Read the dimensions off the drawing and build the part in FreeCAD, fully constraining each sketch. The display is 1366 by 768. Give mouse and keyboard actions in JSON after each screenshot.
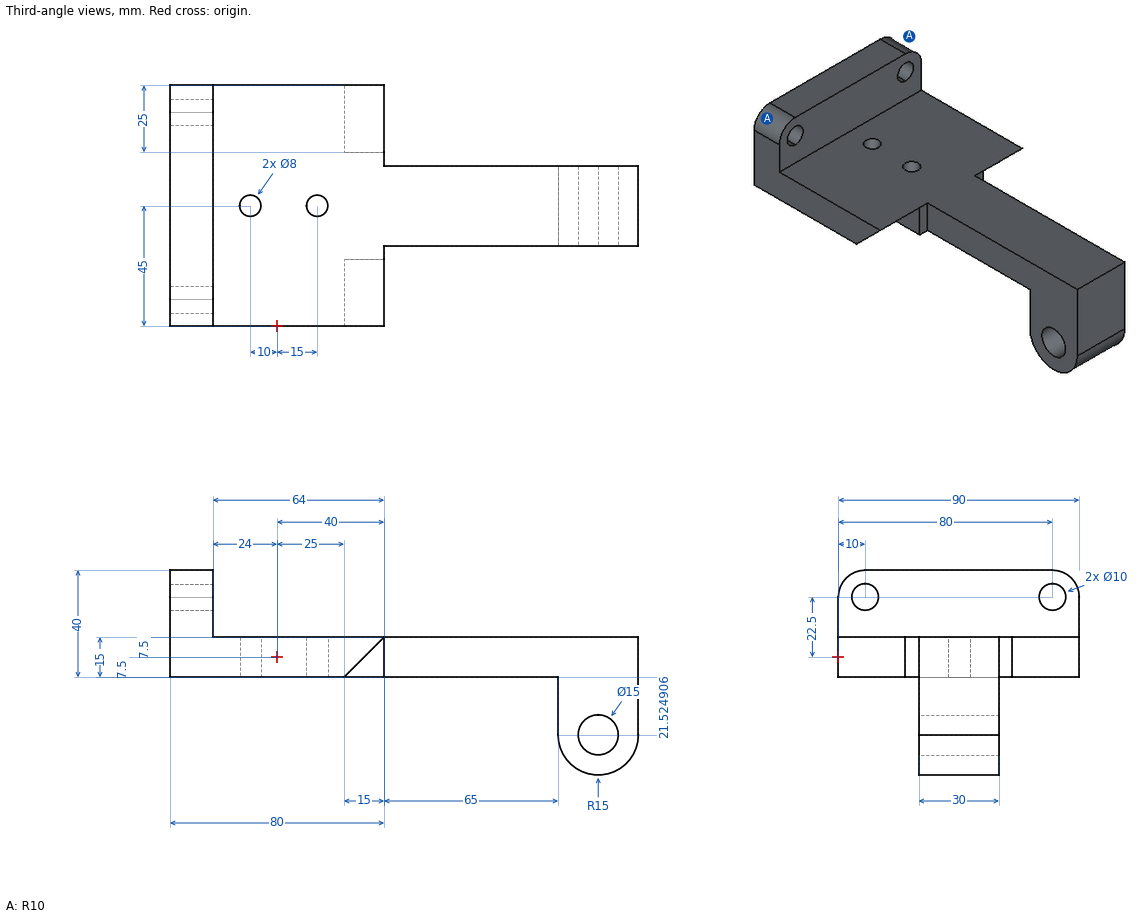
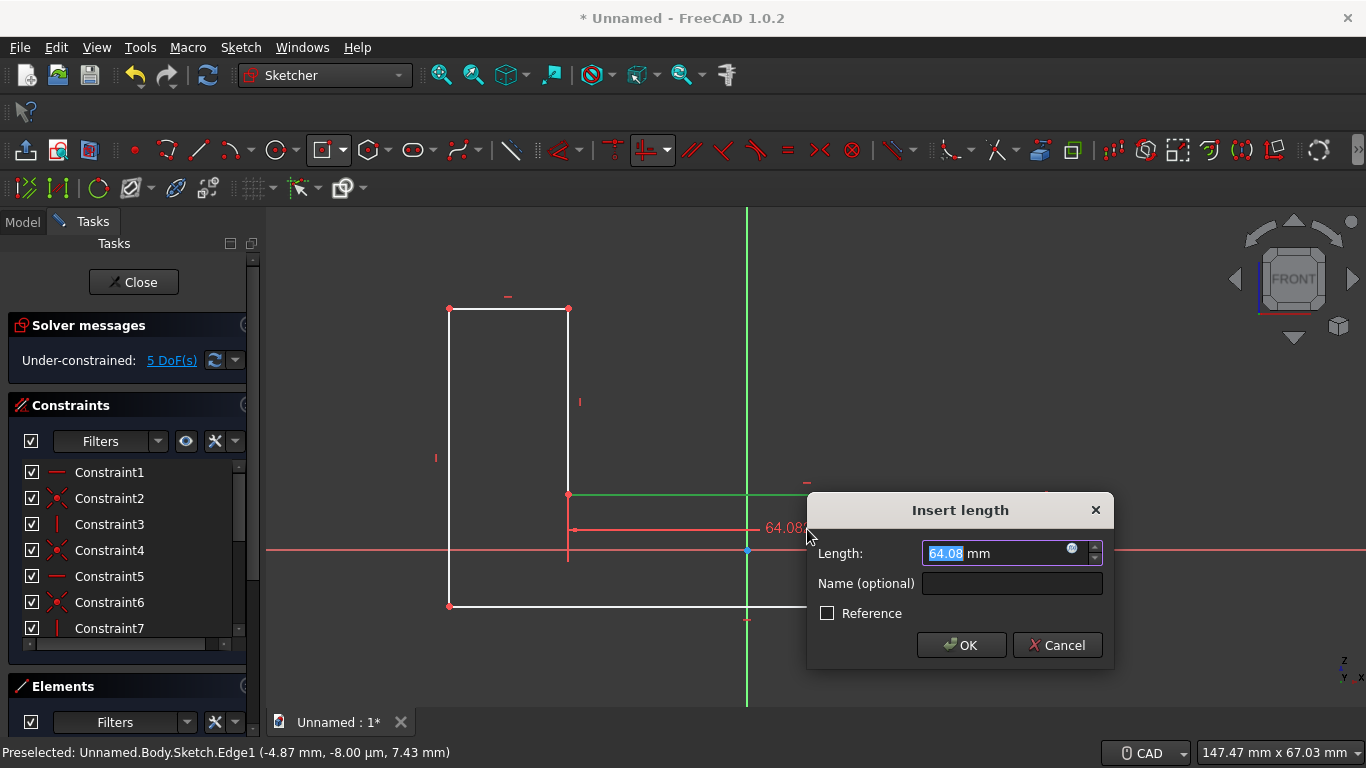
{"action": "type", "text": "64"}
{"action": "key", "text": "Return"}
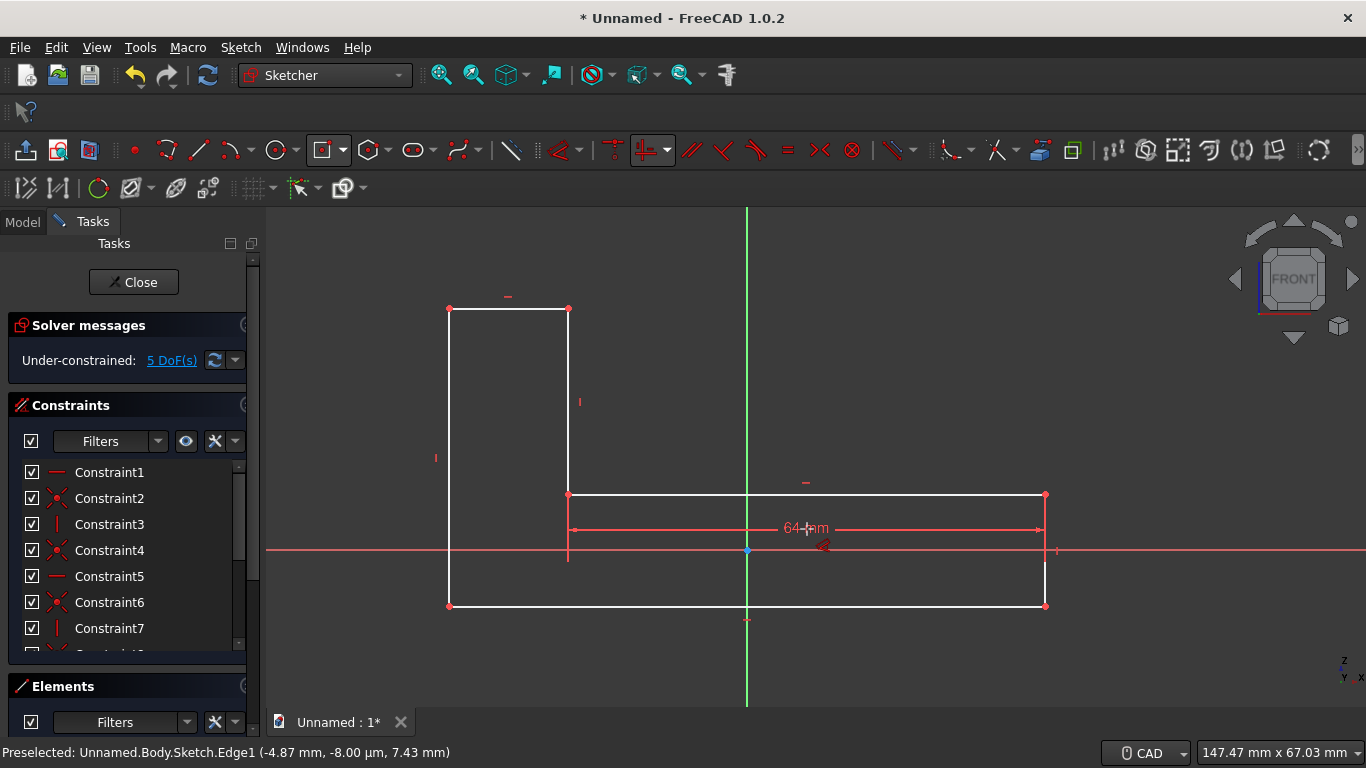
{"action": "left_click", "coordinate": [1045, 529]}
{"action": "left_click", "coordinate": [1079, 525]}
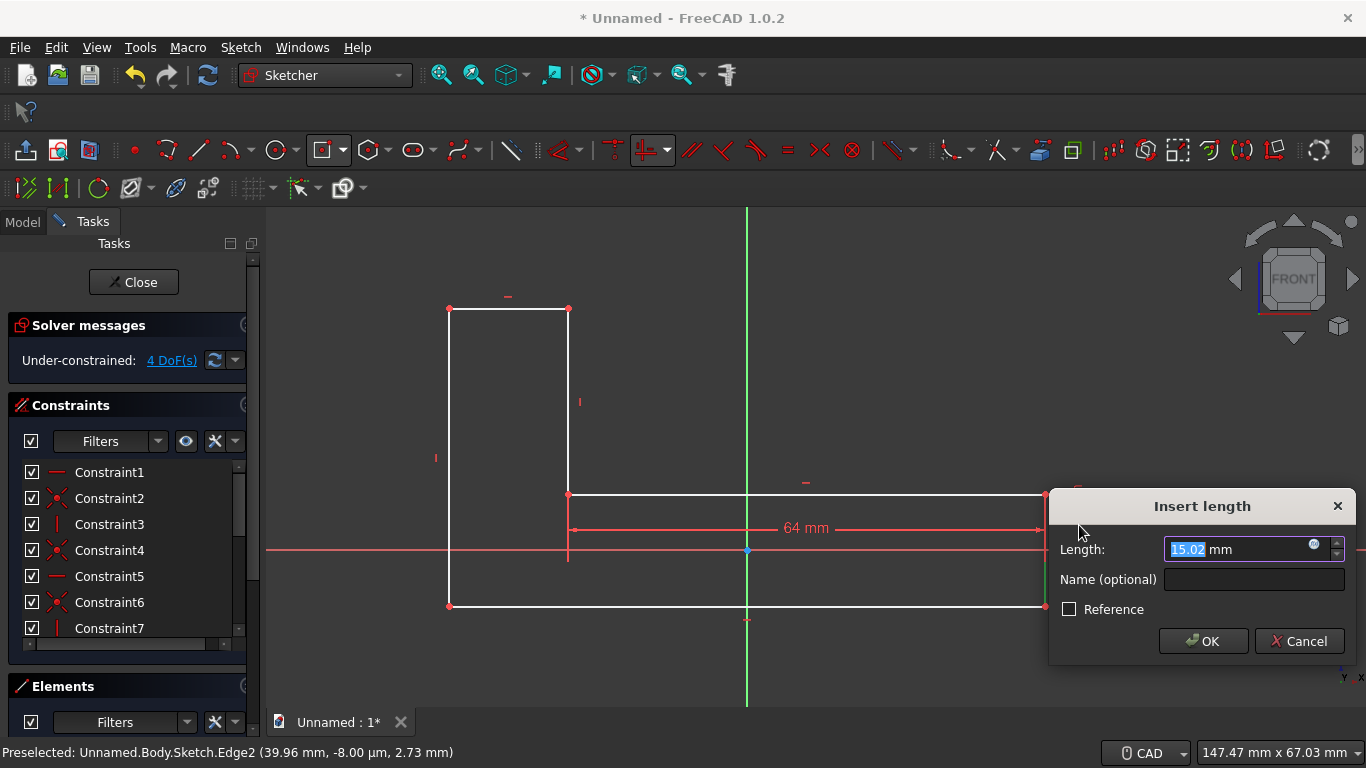
{"action": "type", "text": "15"}
{"action": "key", "text": "Return"}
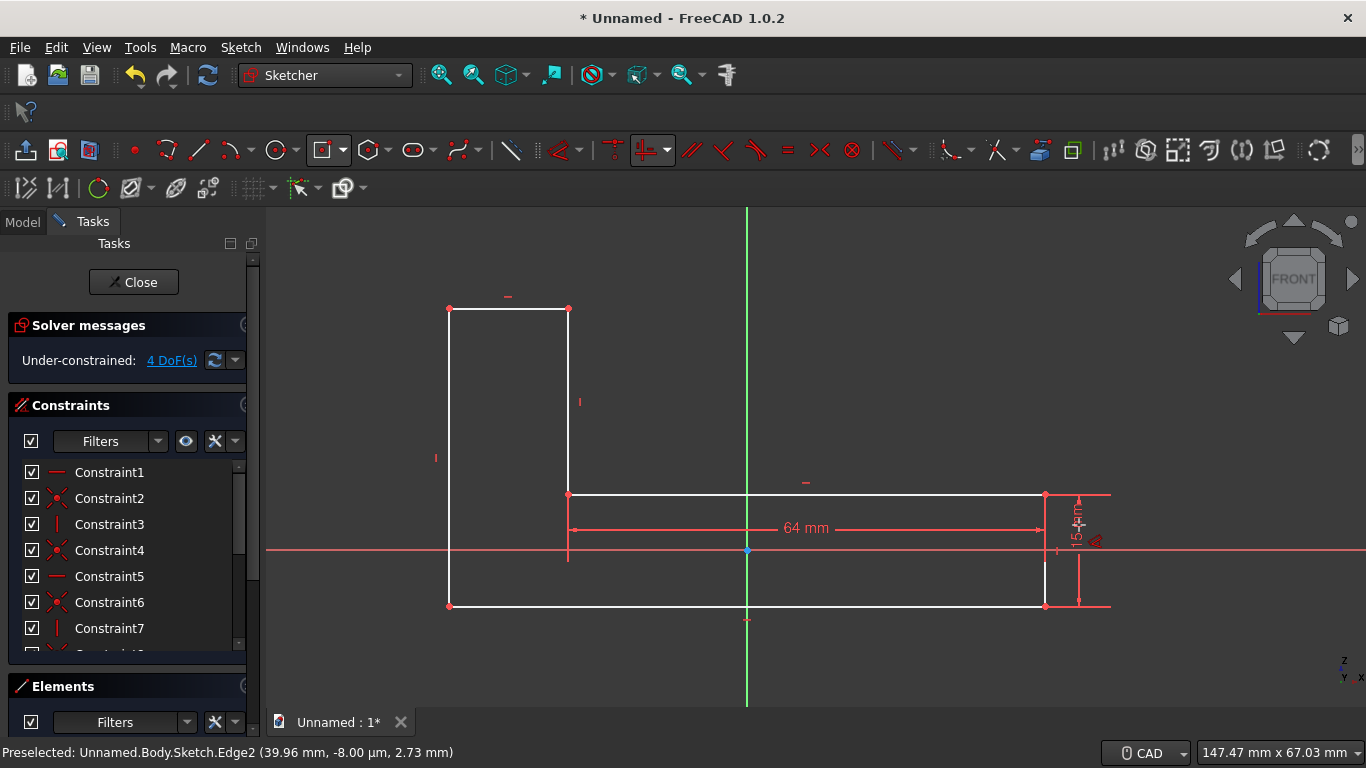
{"action": "left_click", "coordinate": [866, 607]}
{"action": "left_click", "coordinate": [610, 641]}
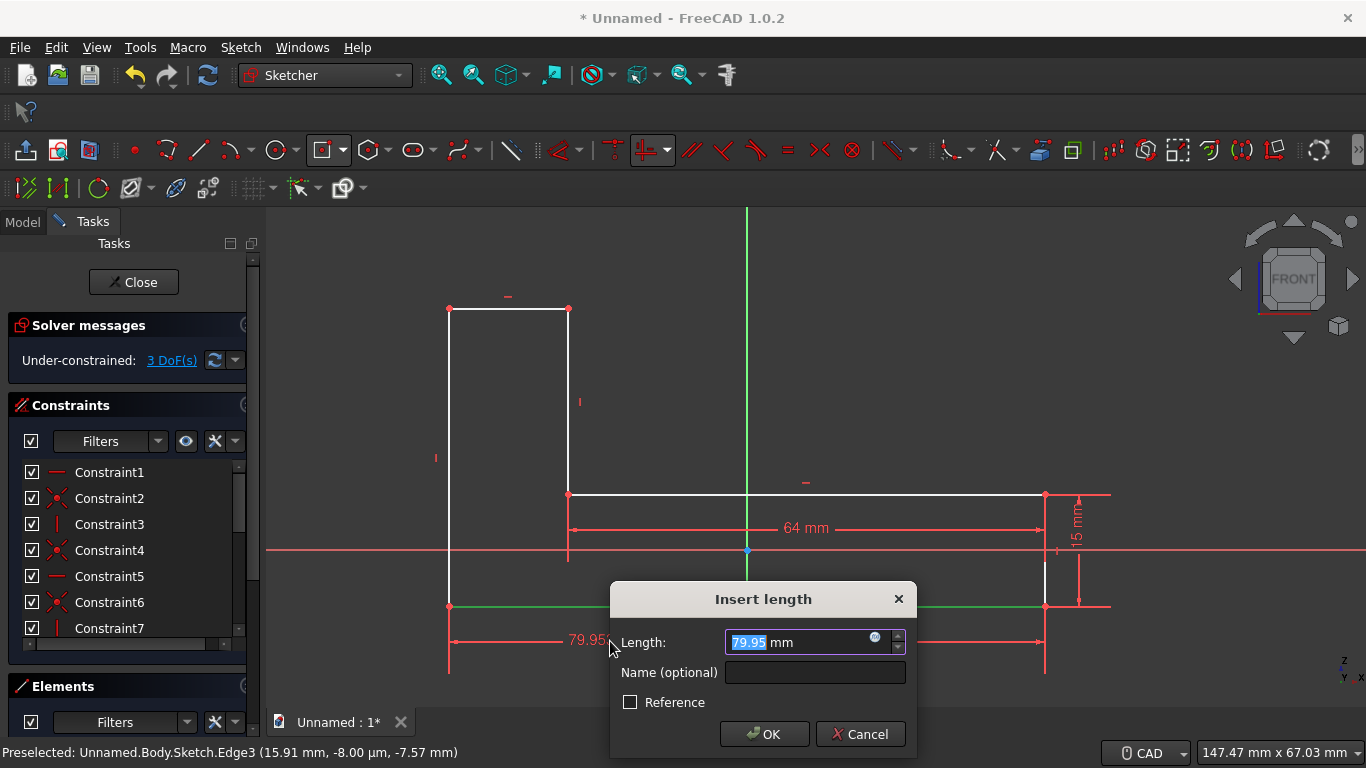
{"action": "type", "text": "80"}
{"action": "key", "text": "Return"}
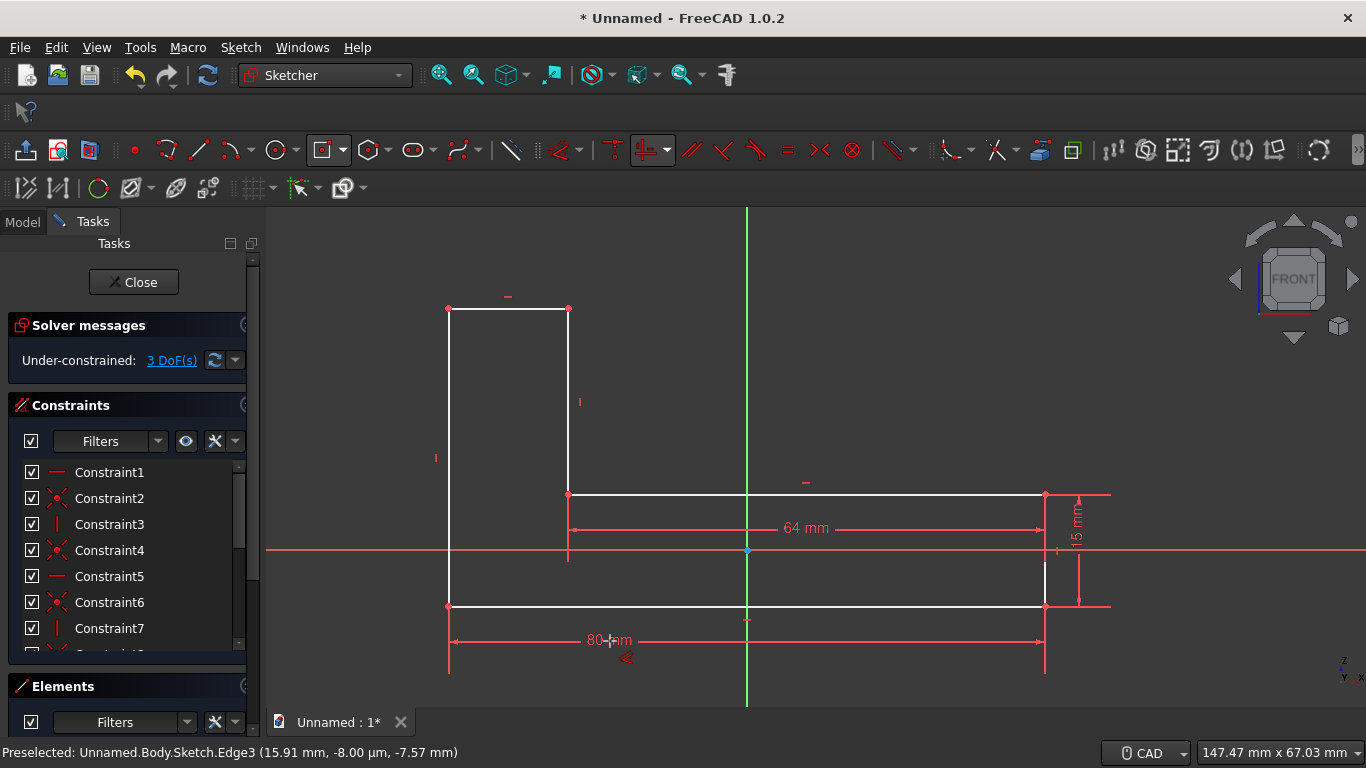
{"action": "left_click", "coordinate": [449, 518]}
{"action": "left_click", "coordinate": [415, 458]}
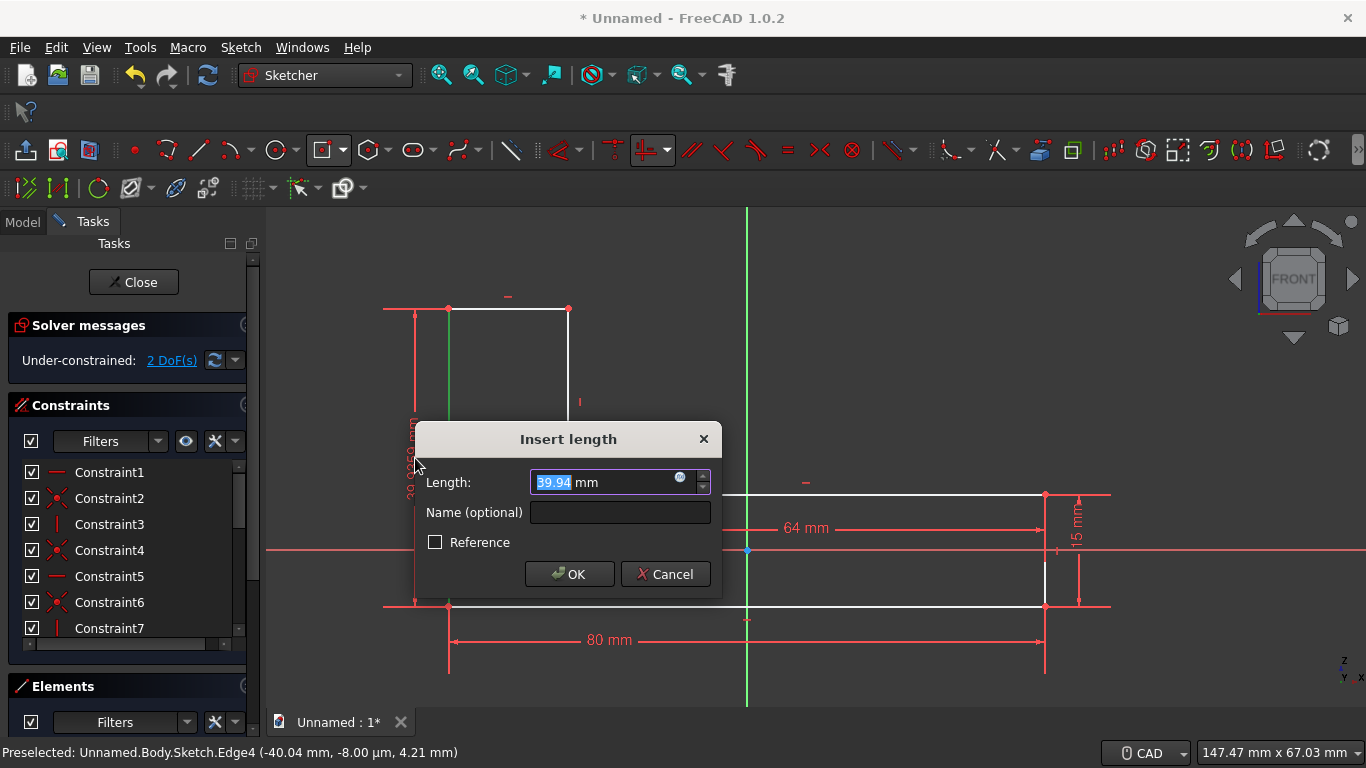
{"action": "type", "text": "40"}
{"action": "key", "text": "Return"}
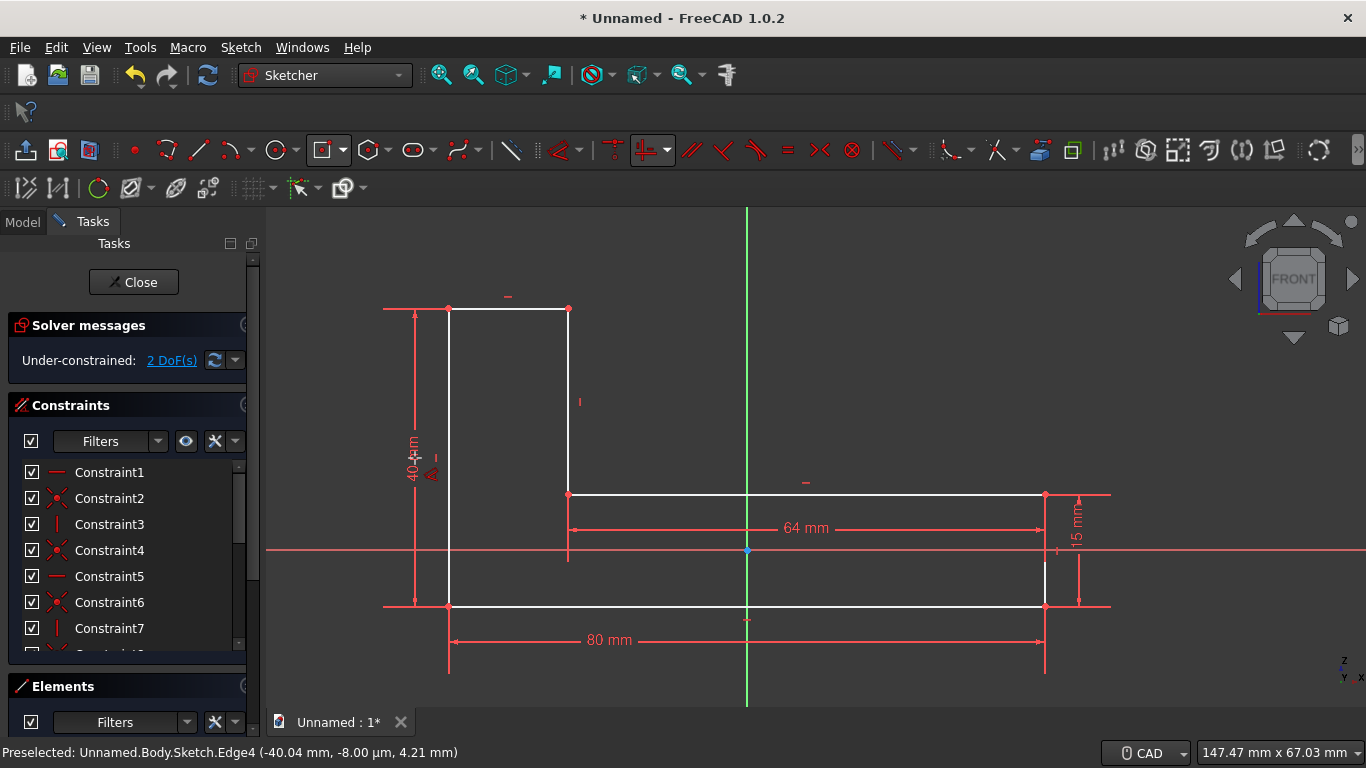
{"action": "left_click", "coordinate": [568, 495]}
{"action": "left_click", "coordinate": [658, 584]}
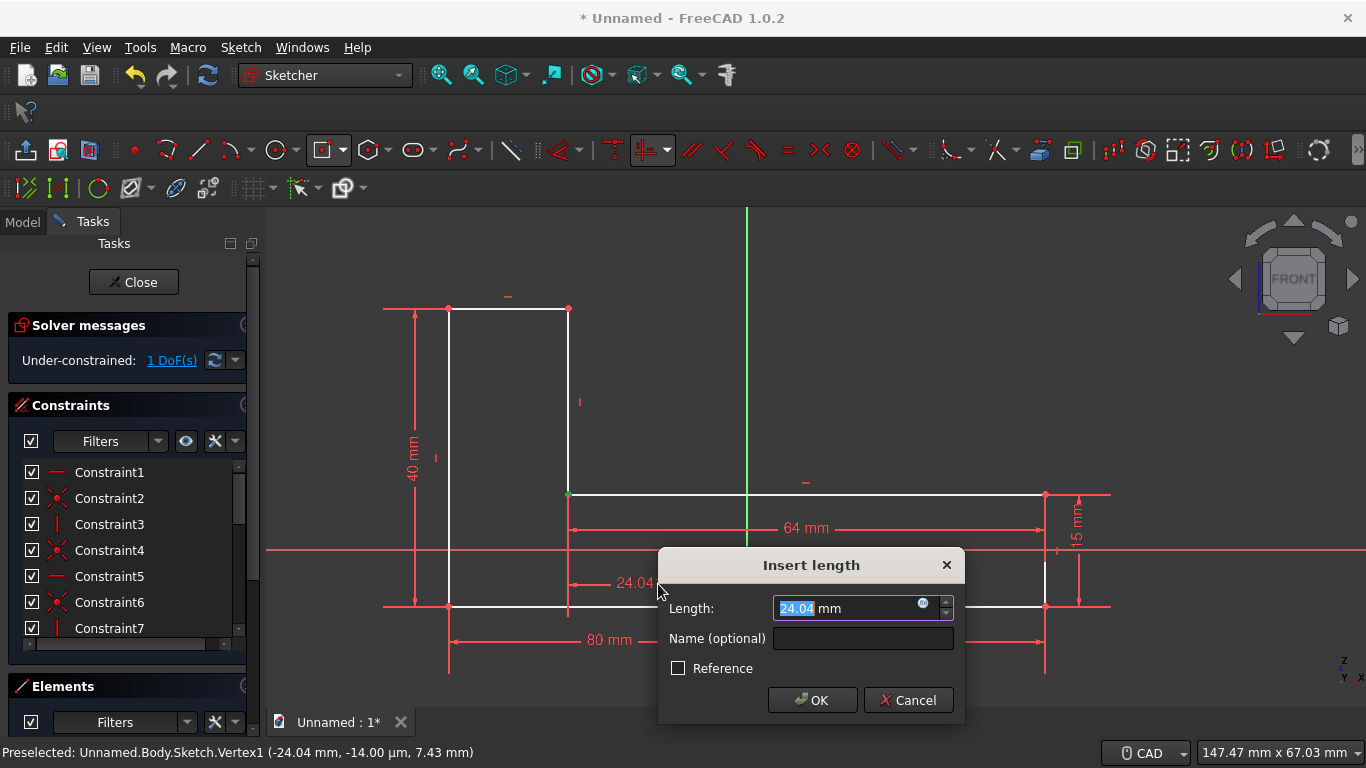
{"action": "type", "text": "24"}
{"action": "key", "text": "Return"}